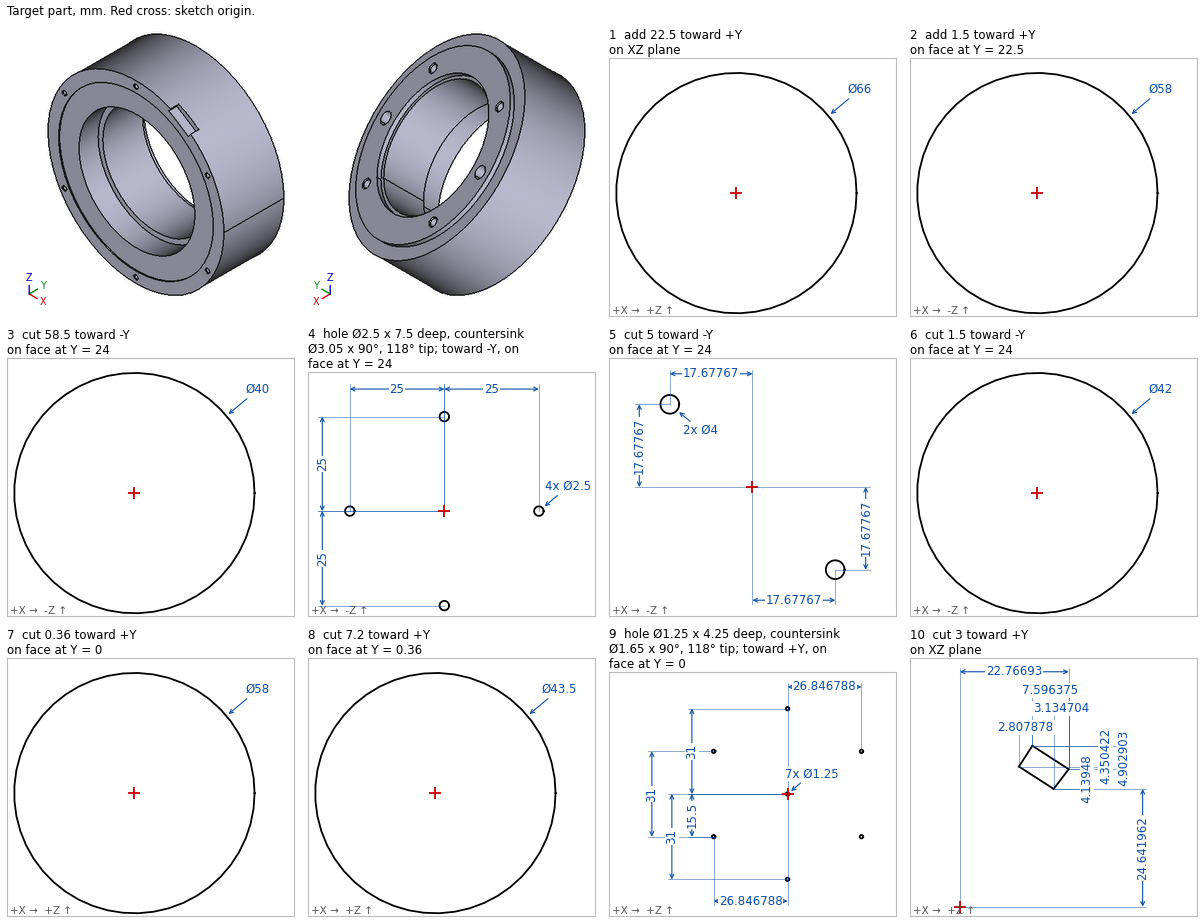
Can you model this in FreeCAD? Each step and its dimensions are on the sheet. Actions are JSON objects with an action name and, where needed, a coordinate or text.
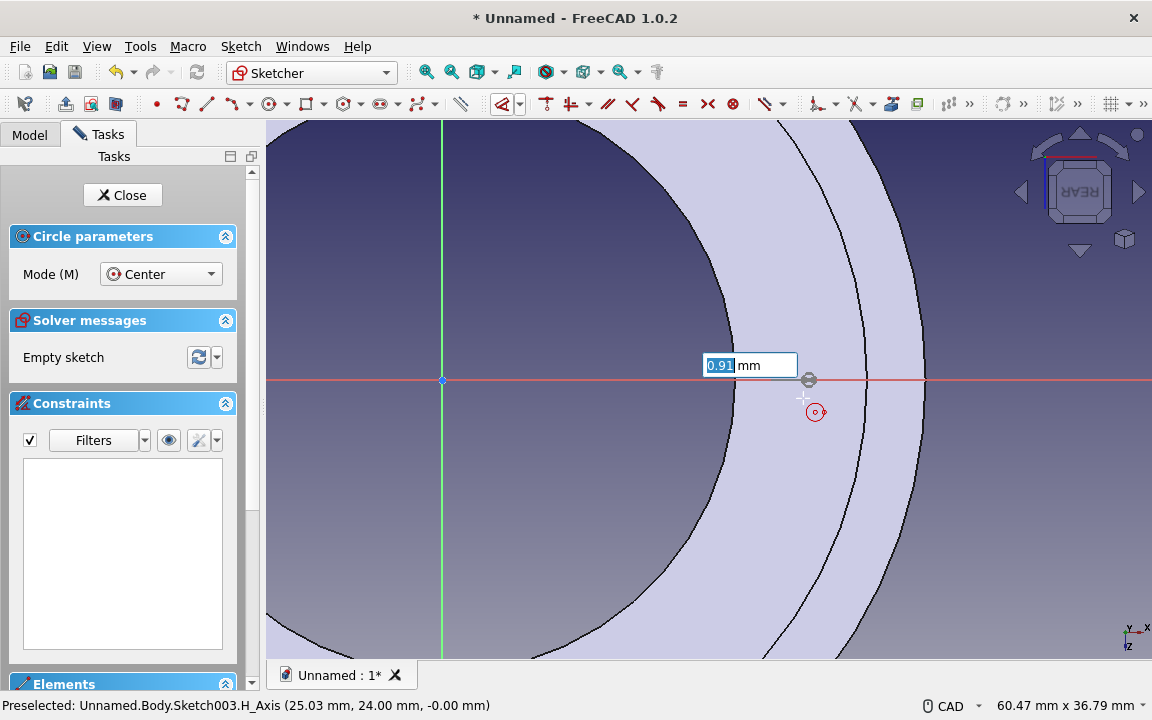
{"action": "left_click", "coordinate": [802, 397]}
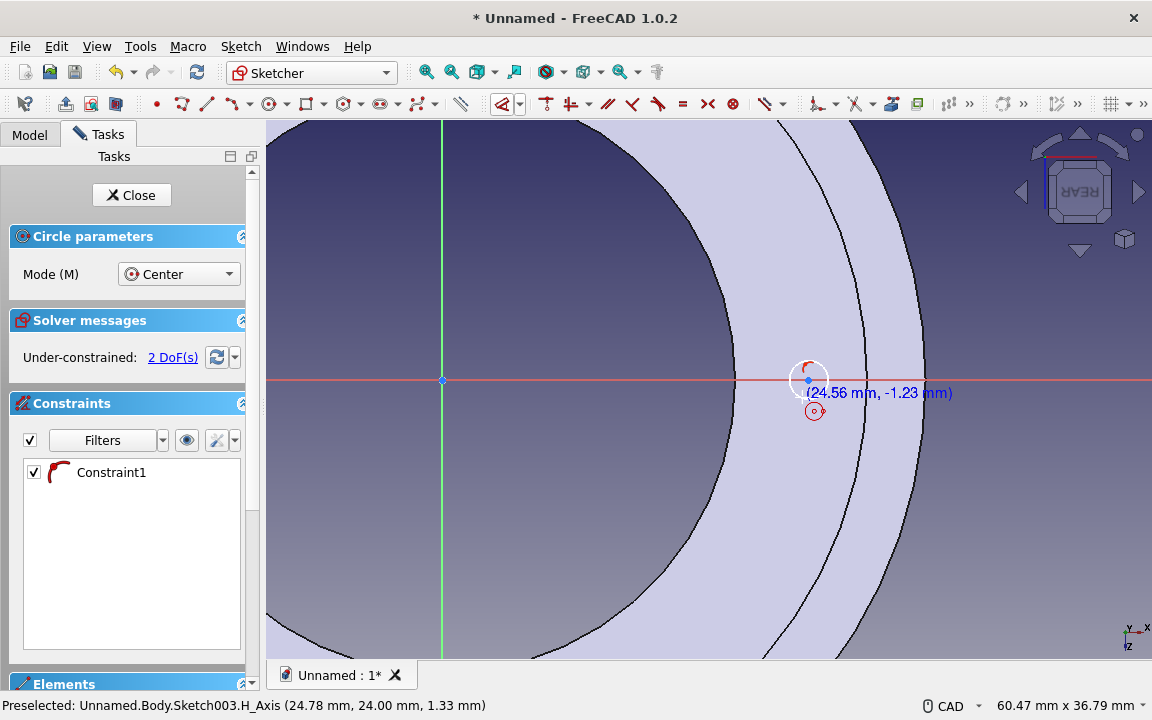
{"action": "scroll", "coordinate": [802, 397], "scroll_direction": "down", "scroll_amount": 4}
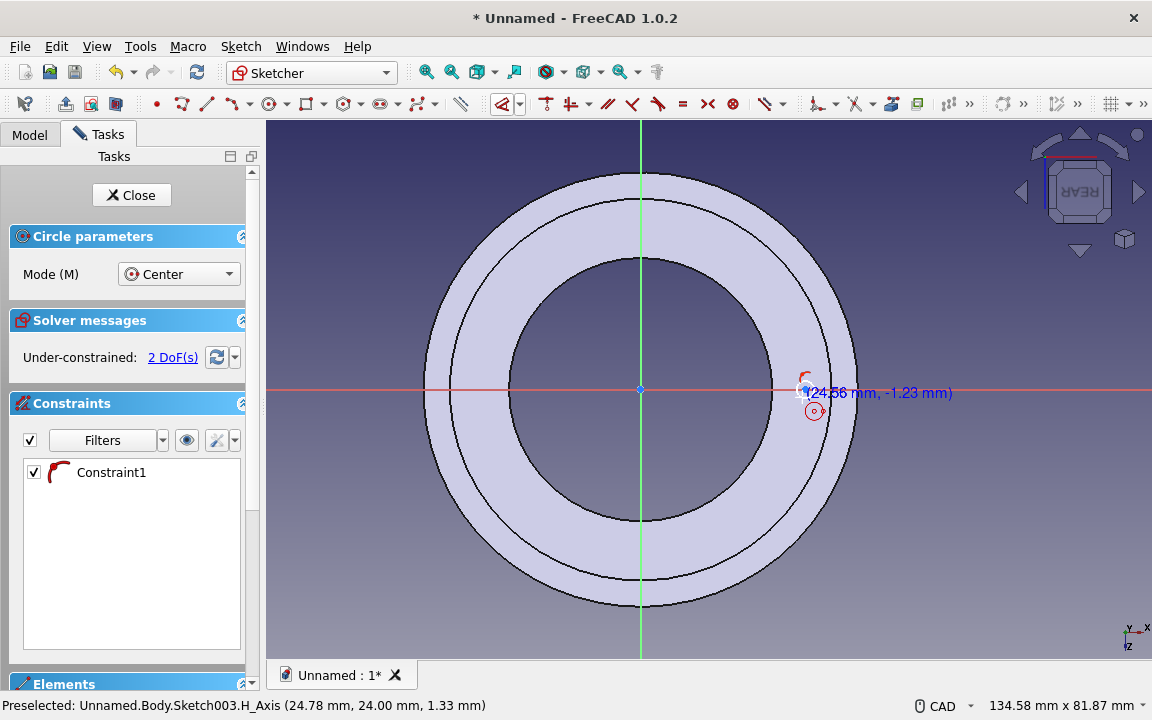
{"action": "scroll", "coordinate": [641, 225], "scroll_direction": "up", "scroll_amount": 6}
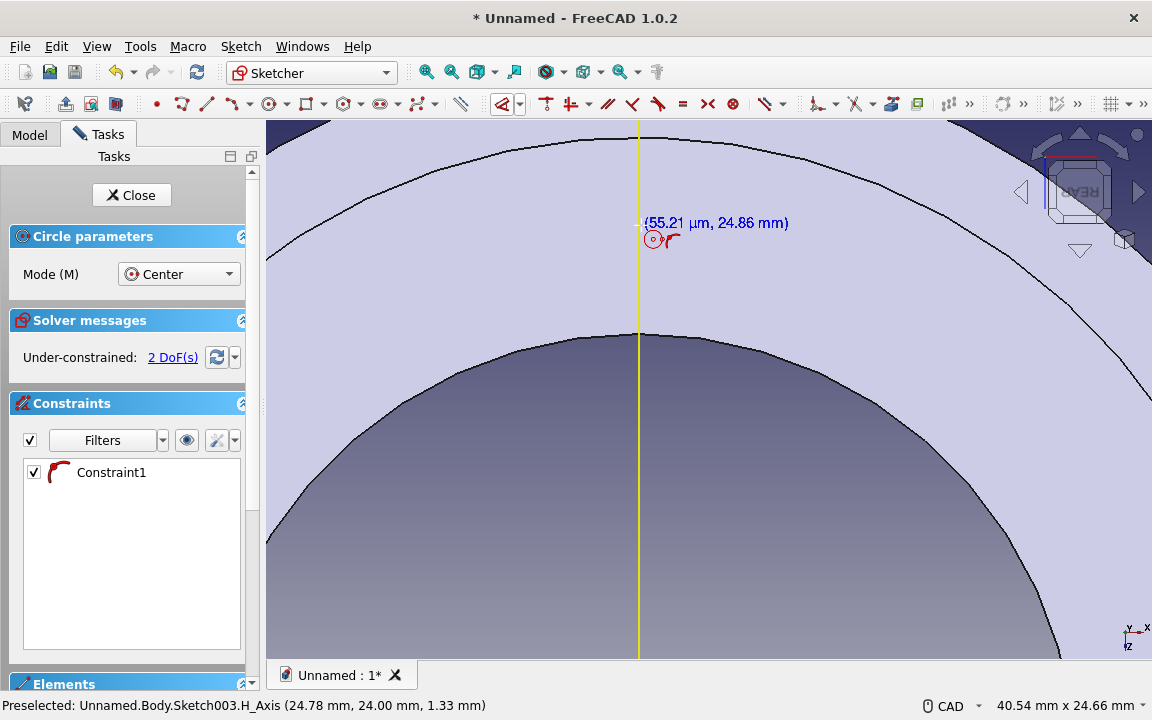
{"action": "scroll", "coordinate": [641, 225], "scroll_direction": "down", "scroll_amount": 6}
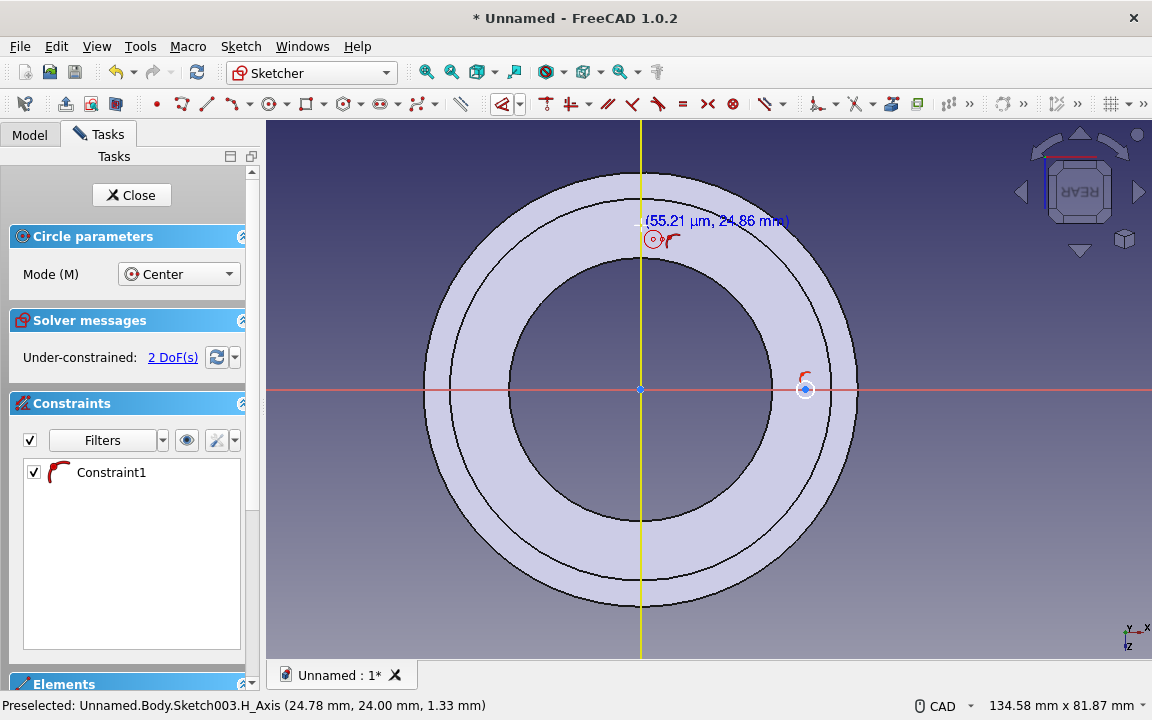
{"action": "left_click", "coordinate": [641, 225]}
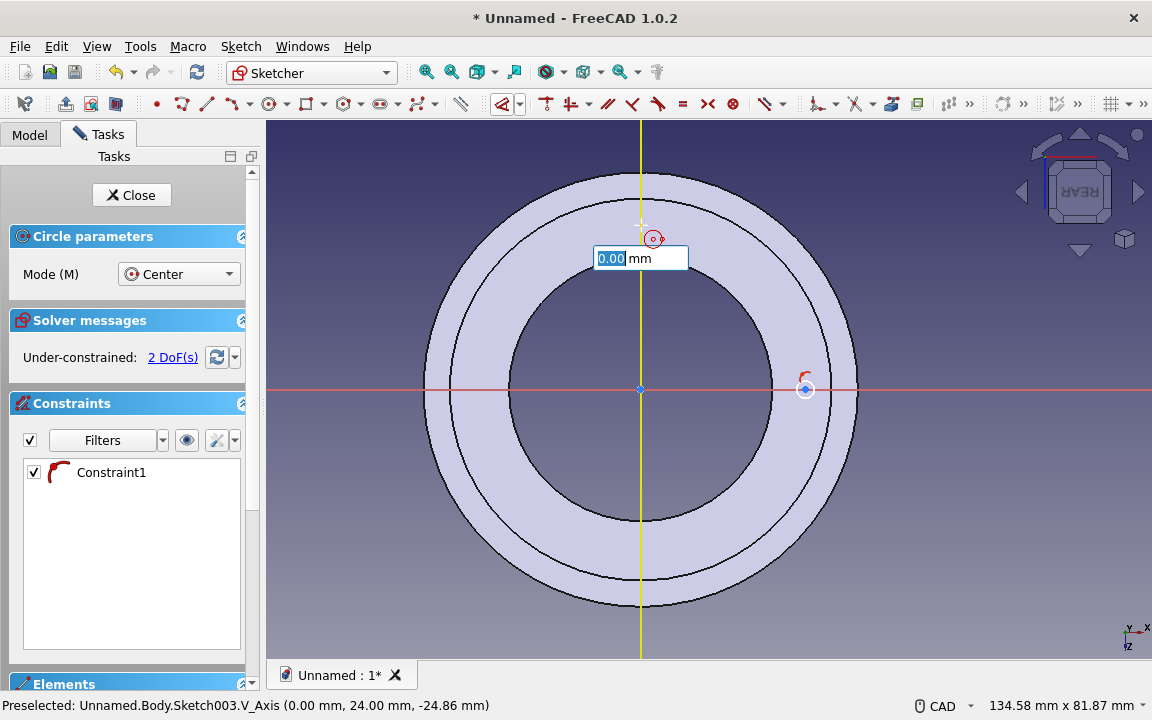
{"action": "scroll", "coordinate": [648, 222], "scroll_direction": "up", "scroll_amount": 4}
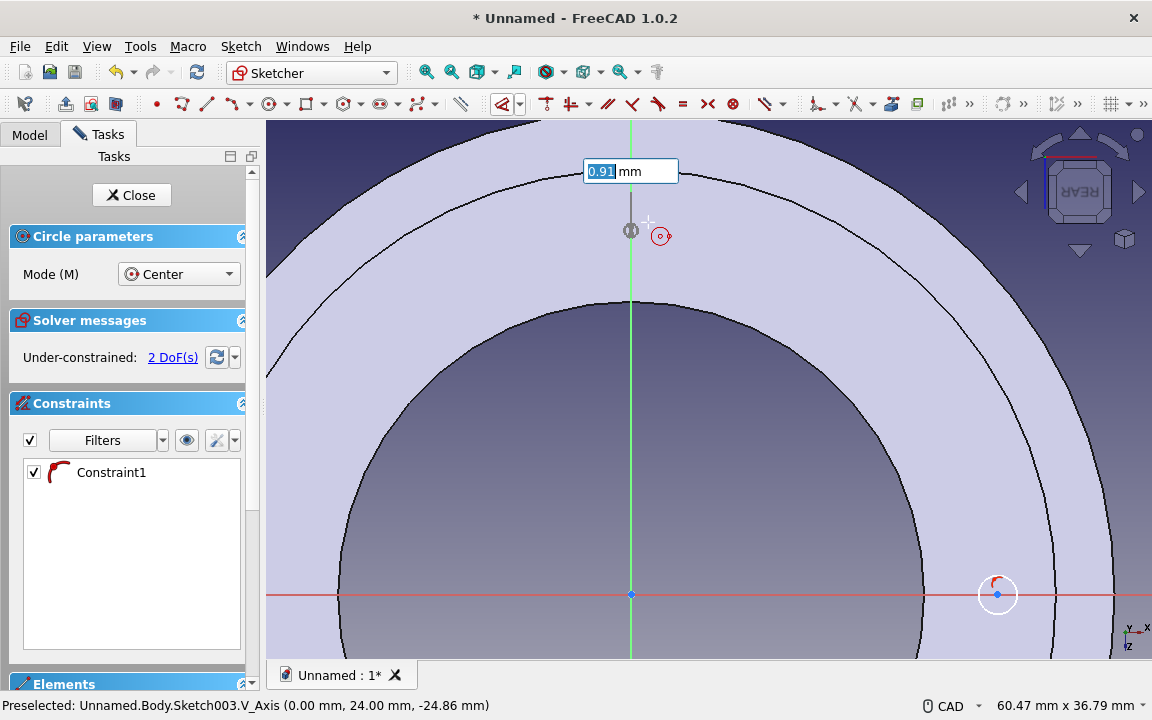
{"action": "left_click", "coordinate": [648, 222]}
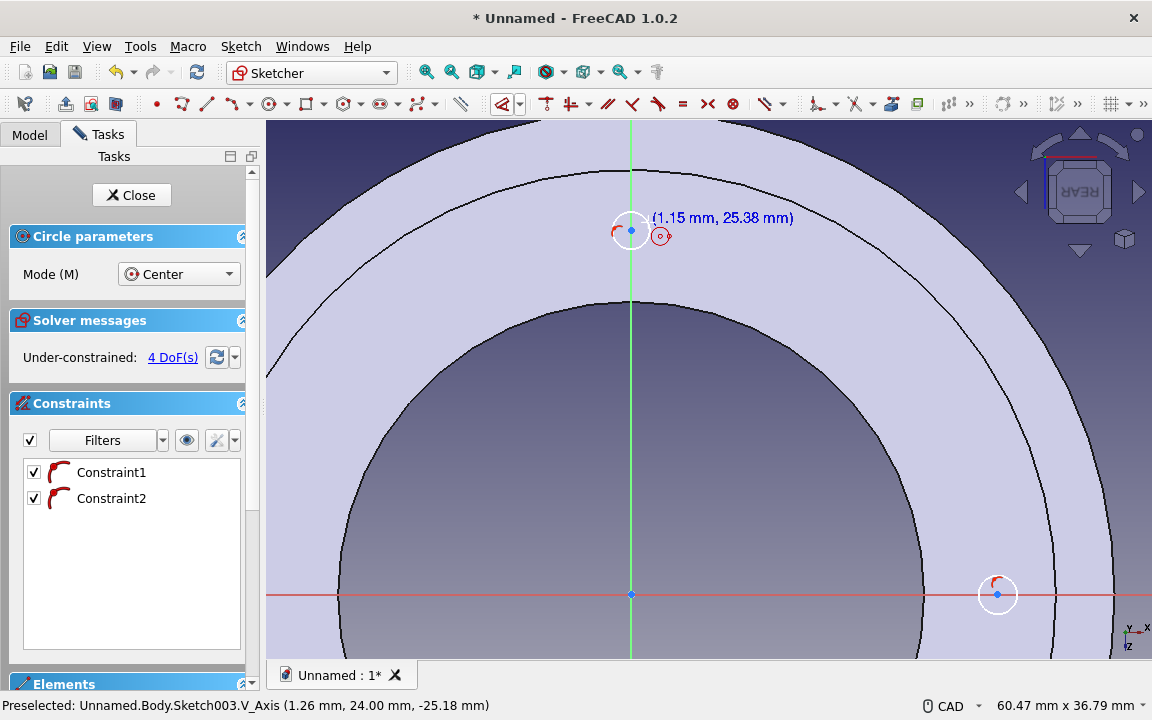
{"action": "scroll", "coordinate": [648, 222], "scroll_direction": "down", "scroll_amount": 4}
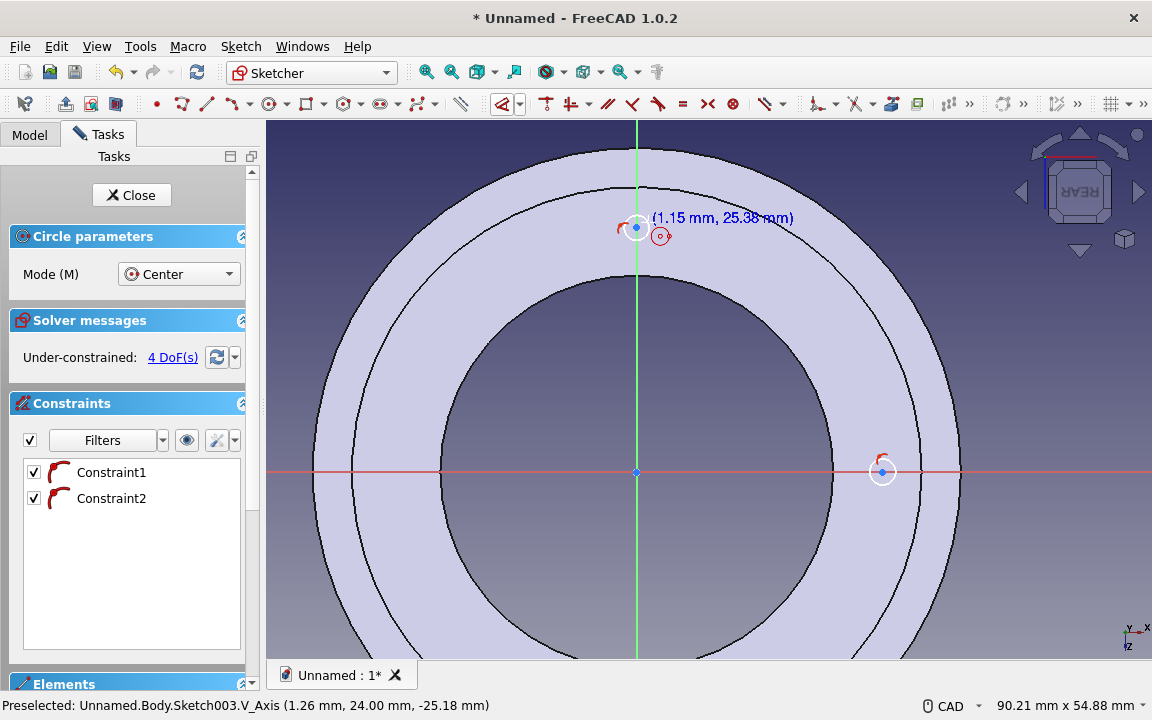
{"action": "scroll", "coordinate": [476, 390], "scroll_direction": "up", "scroll_amount": 6}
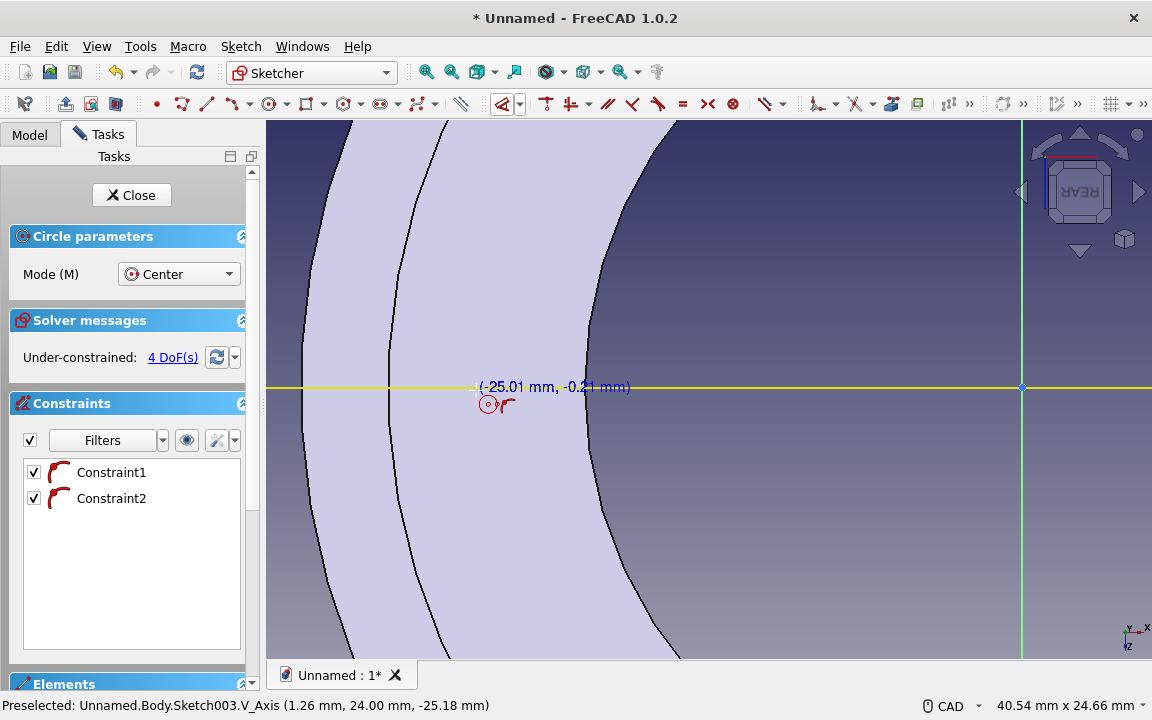
{"action": "scroll", "coordinate": [476, 390], "scroll_direction": "down", "scroll_amount": 6}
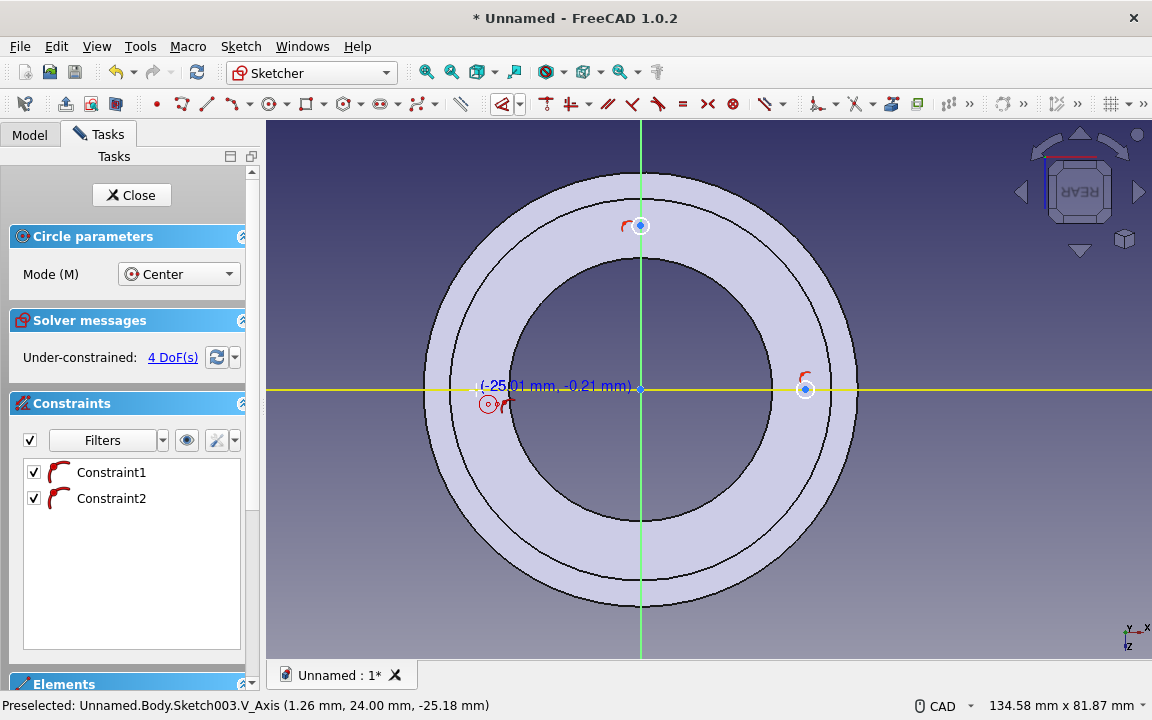
{"action": "left_click", "coordinate": [476, 390]}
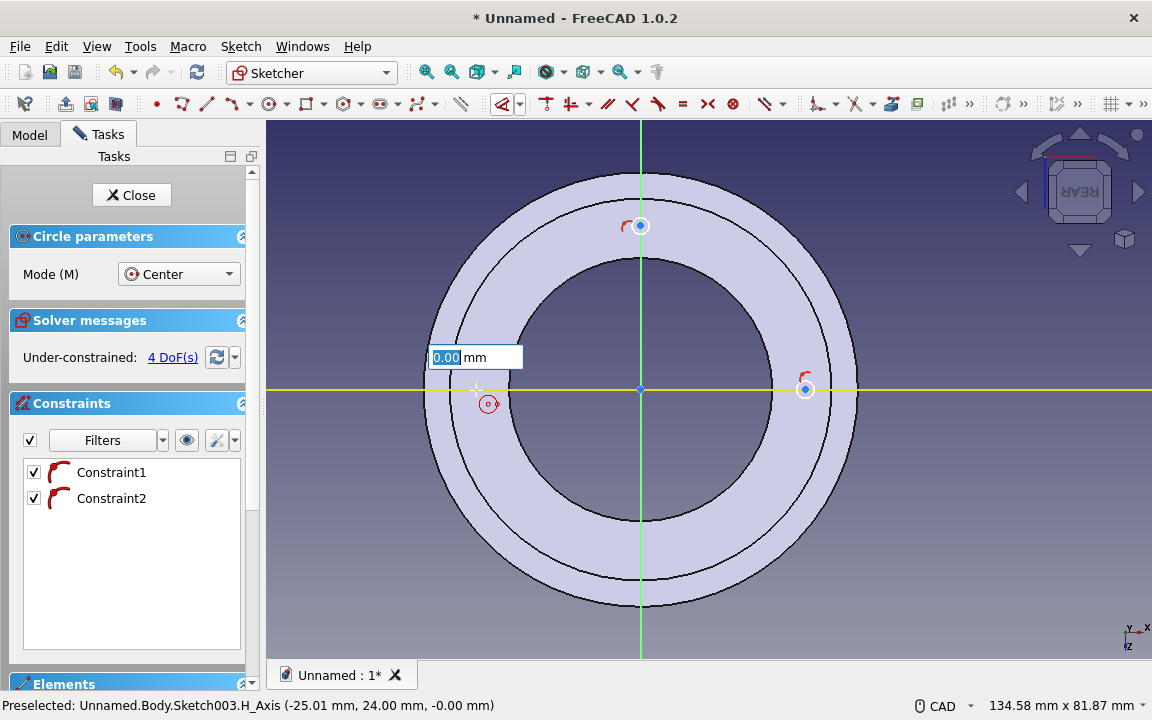
{"action": "scroll", "coordinate": [473, 397], "scroll_direction": "up", "scroll_amount": 4}